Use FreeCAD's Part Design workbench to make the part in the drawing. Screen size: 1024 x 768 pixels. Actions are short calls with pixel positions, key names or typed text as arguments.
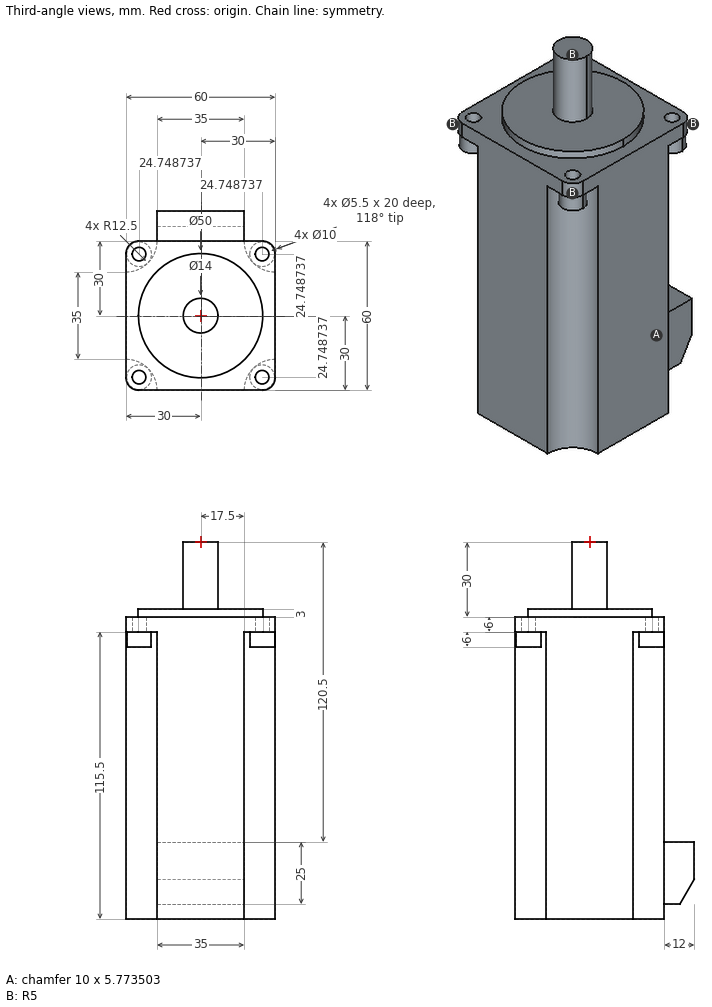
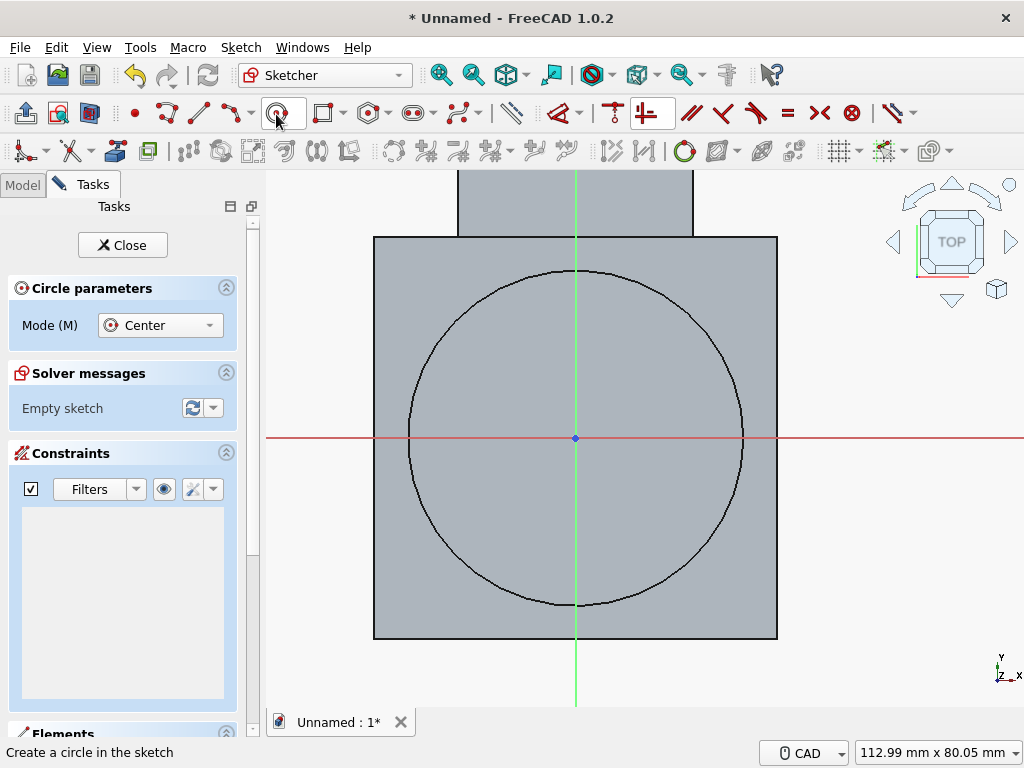
scroll(742, 272, up, 2)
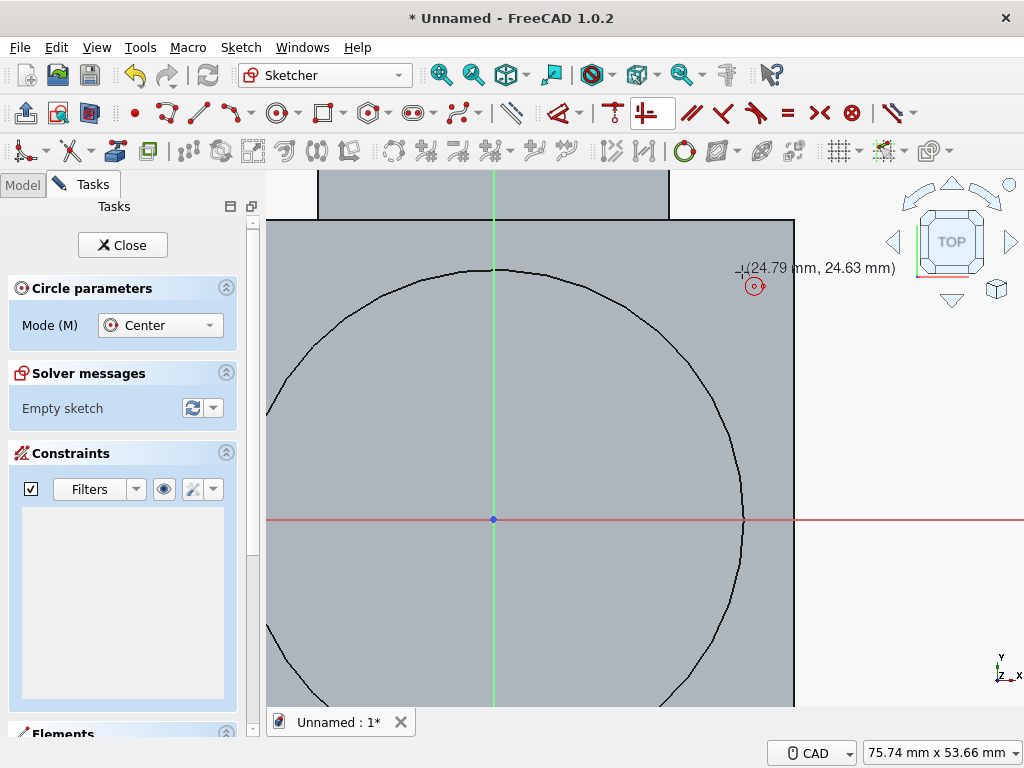
click(741, 272)
click(761, 253)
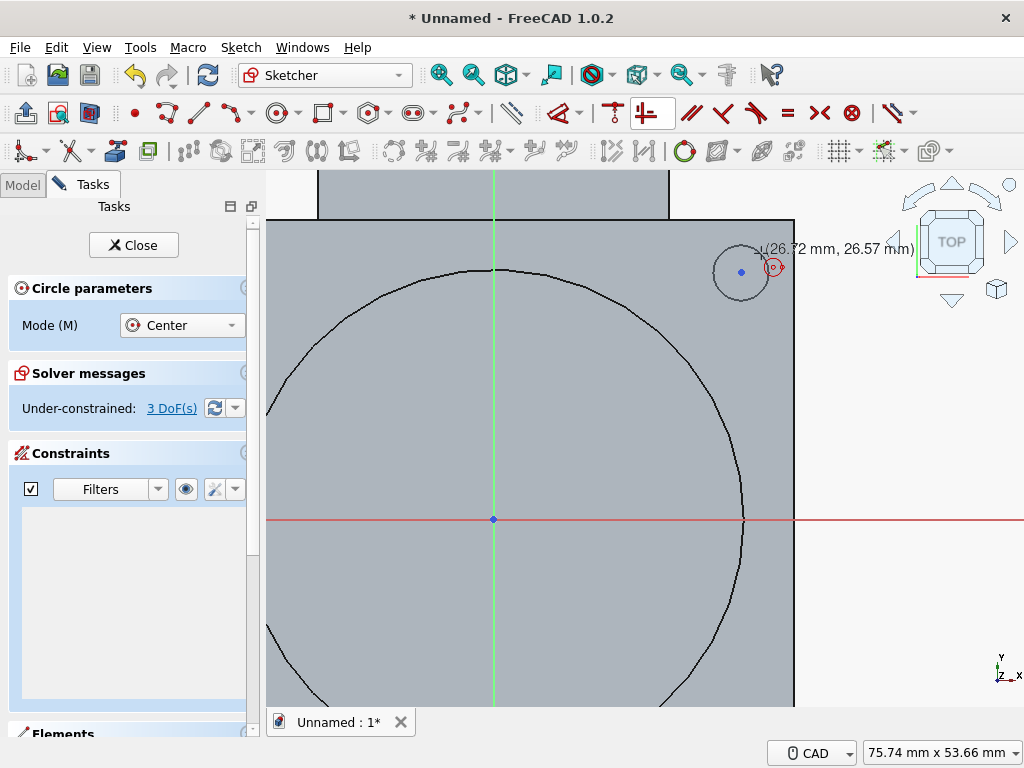
scroll(745, 273, down, 2)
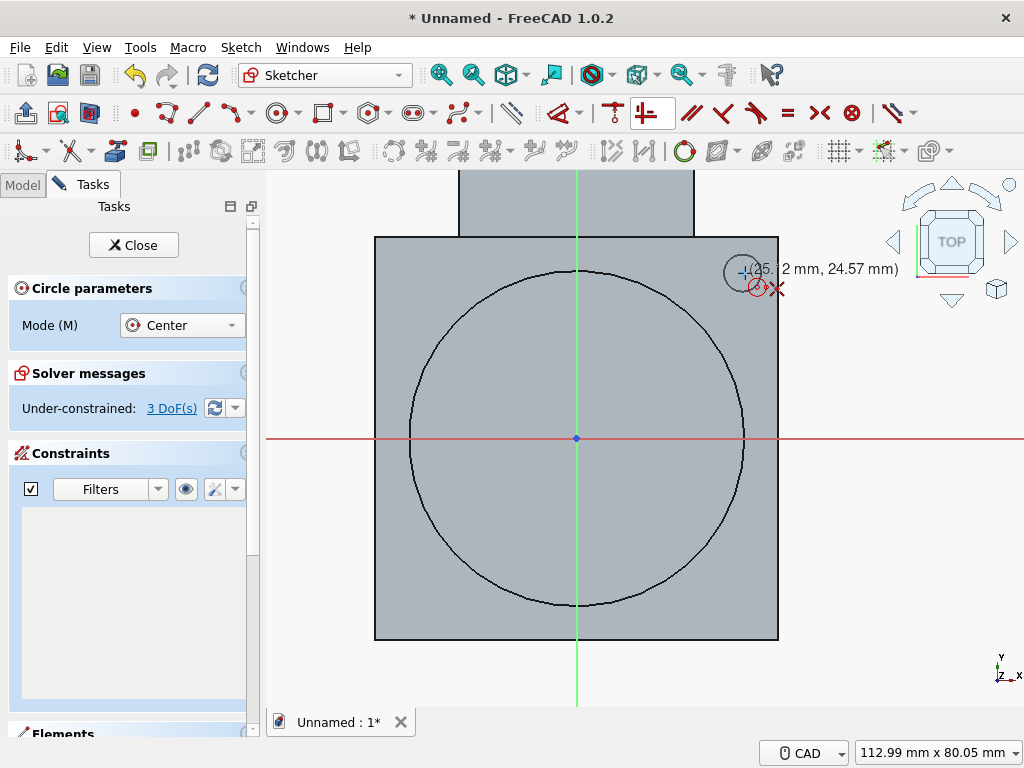
scroll(411, 273, up, 2)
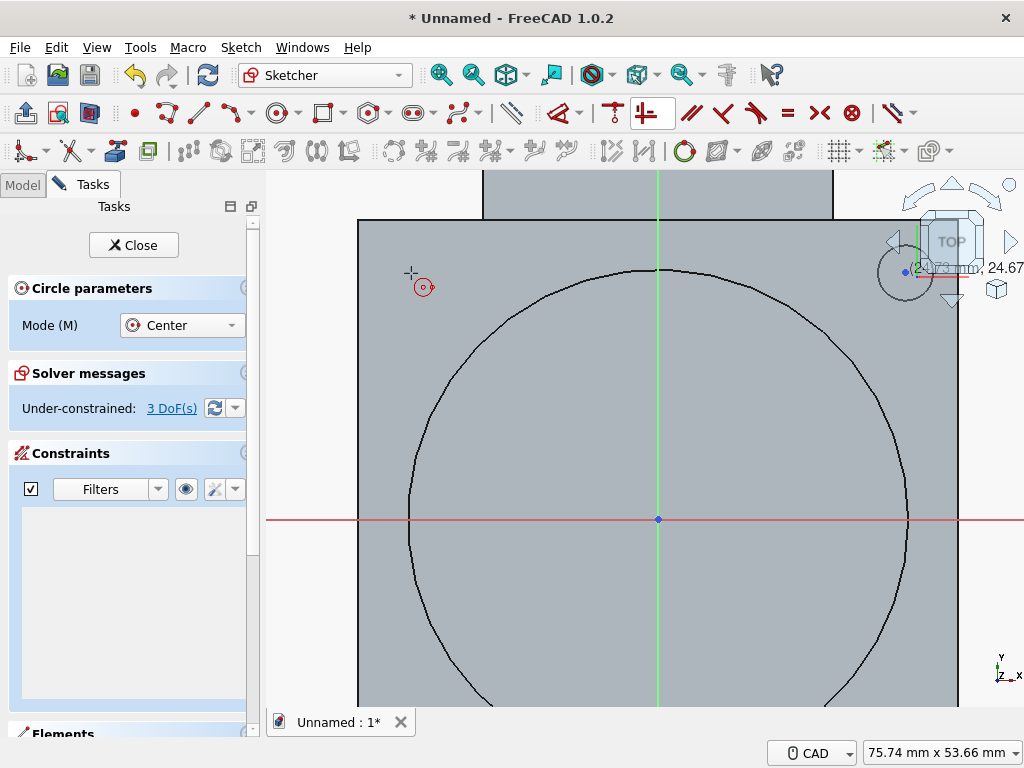
click(410, 272)
click(430, 253)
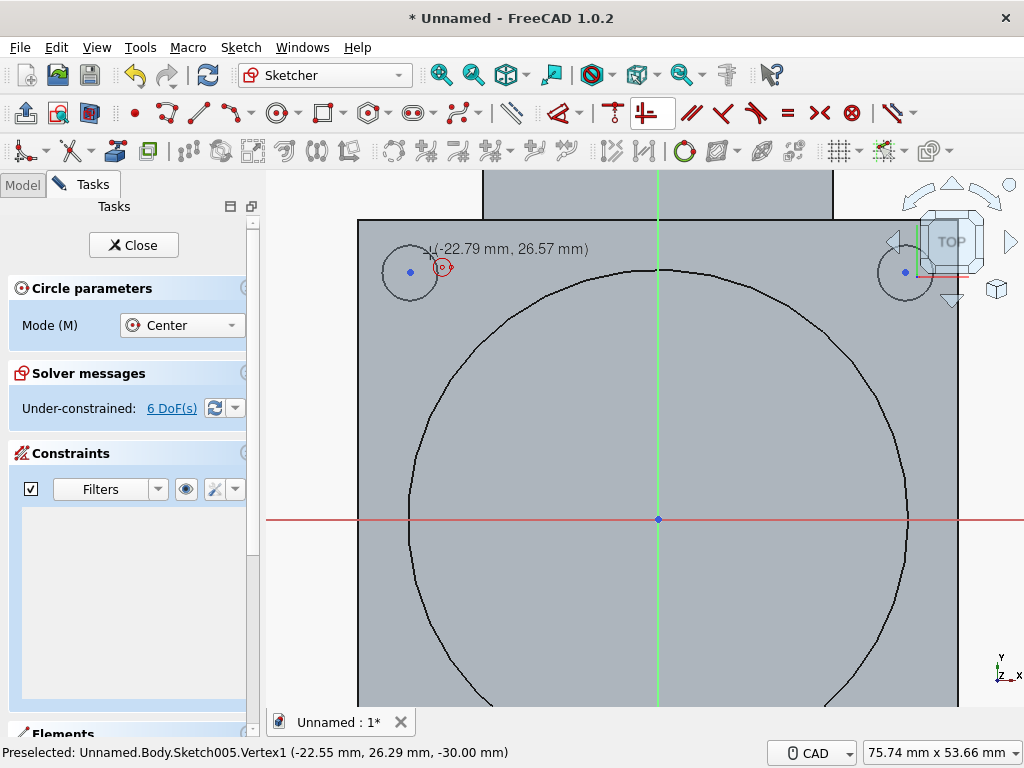
scroll(411, 273, down, 2)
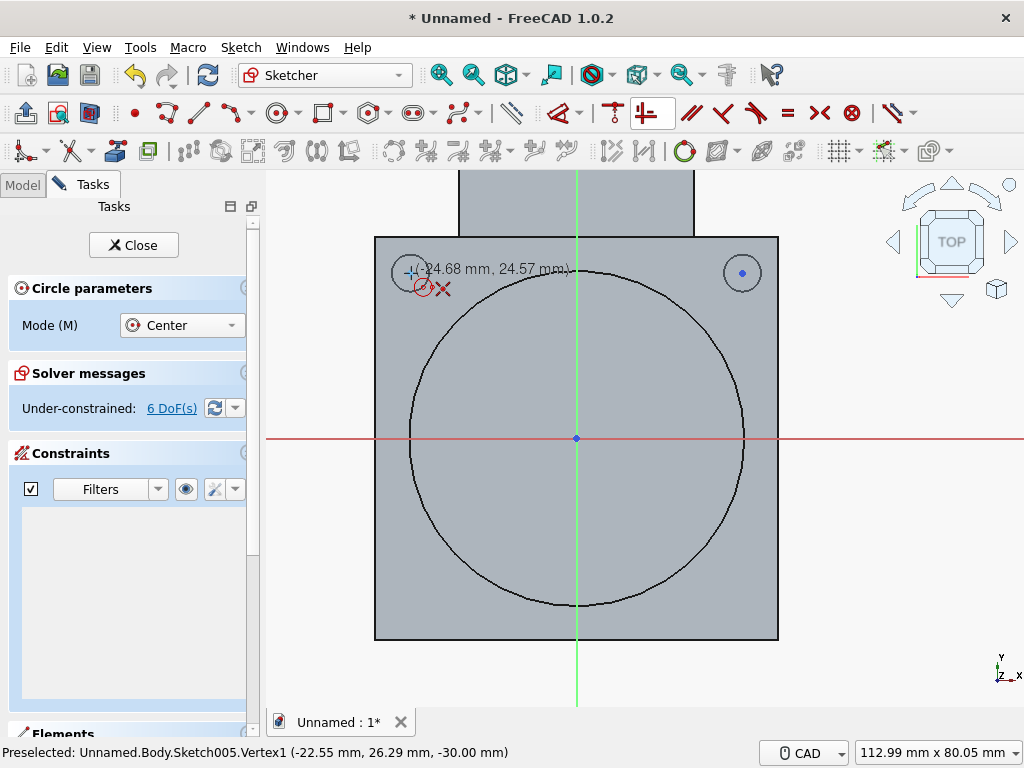
scroll(743, 605, up, 2)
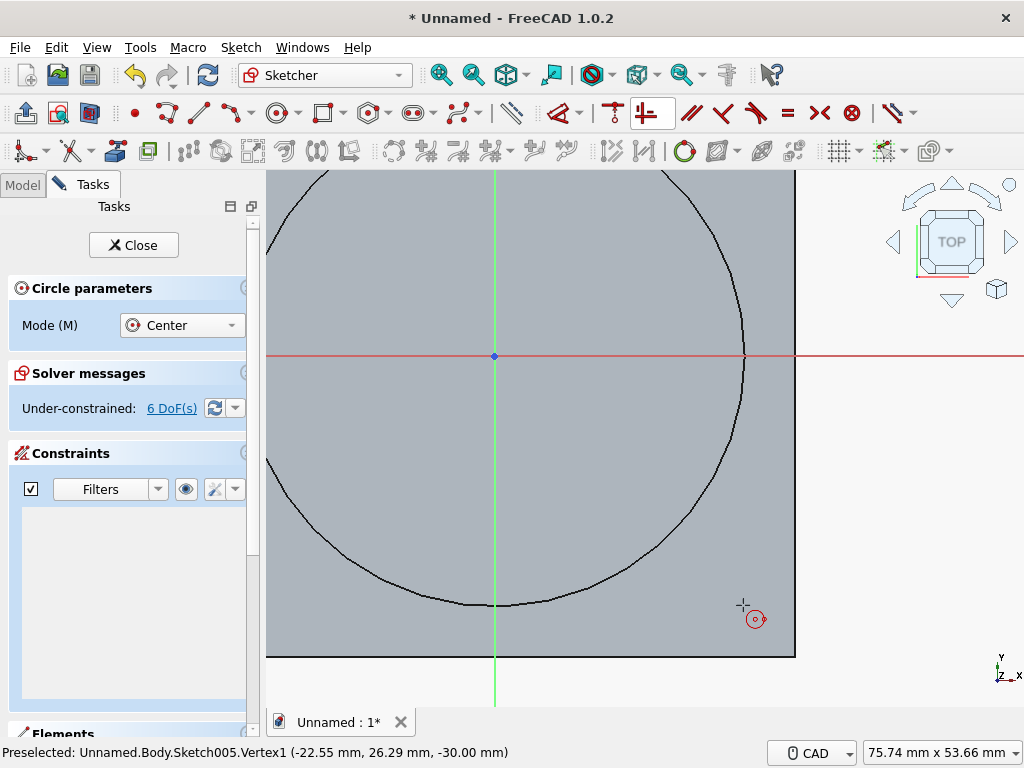
click(742, 604)
click(762, 585)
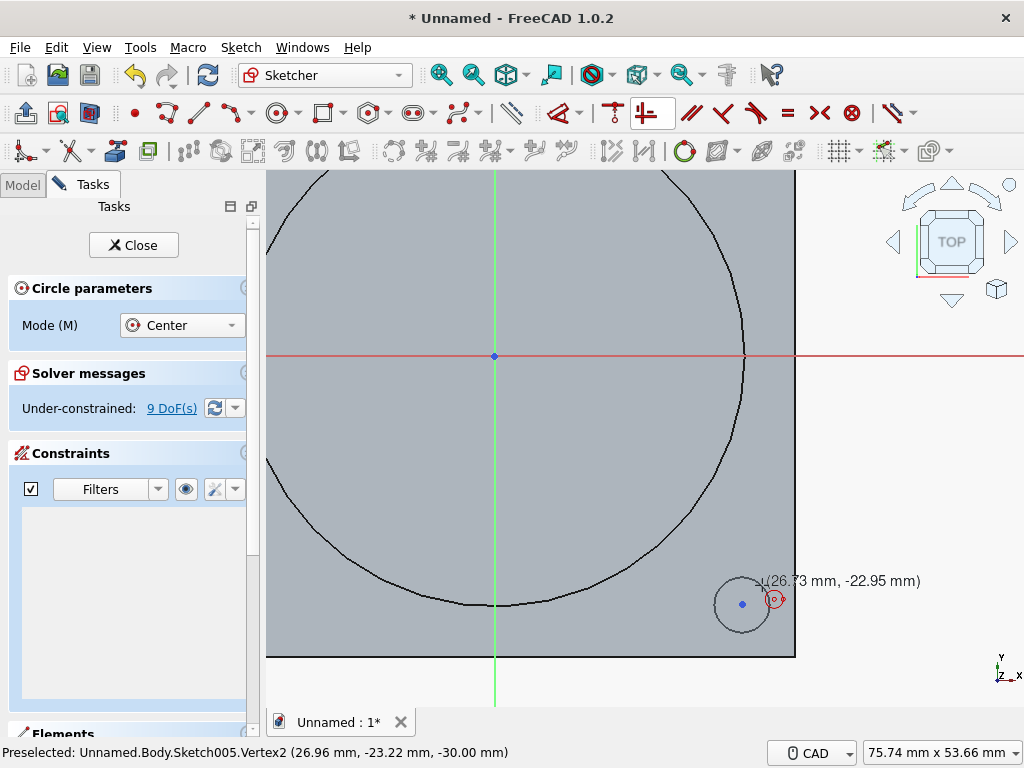
scroll(743, 606, down, 2)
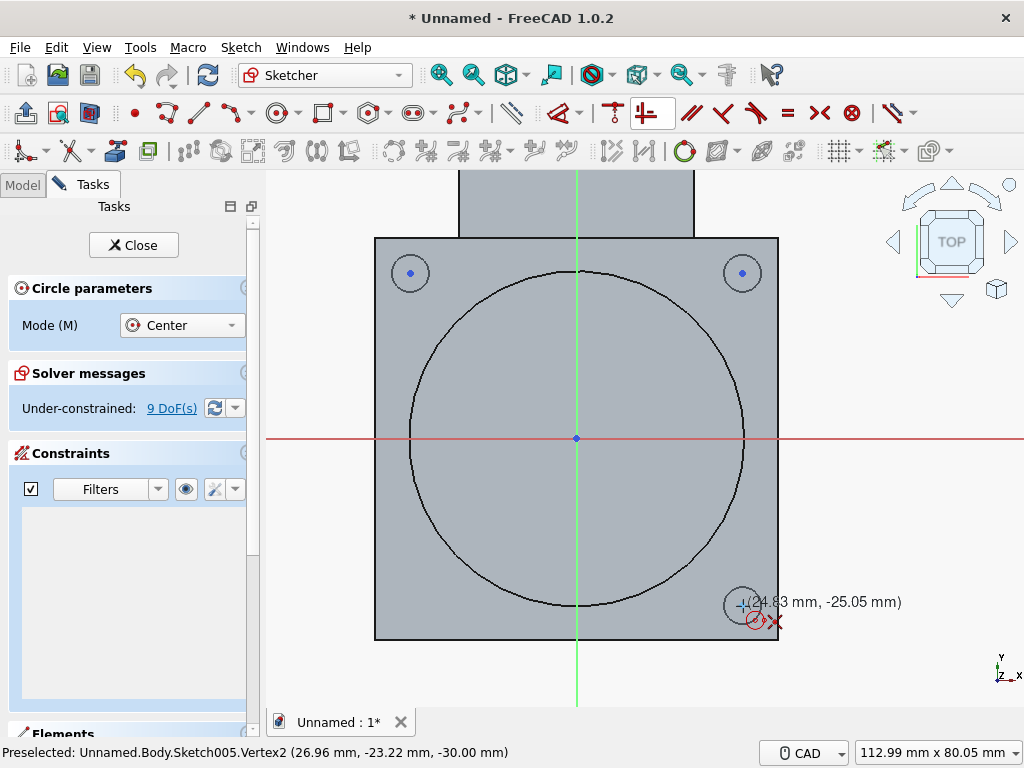
scroll(411, 605, up, 2)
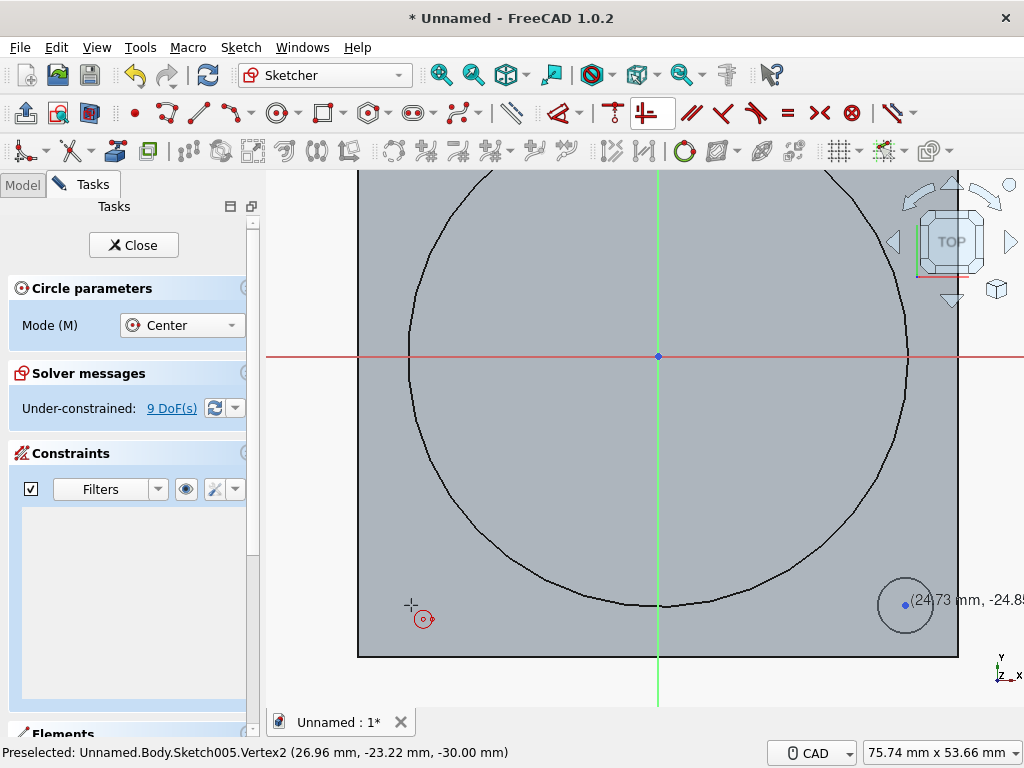
click(410, 604)
click(430, 585)
key(Escape)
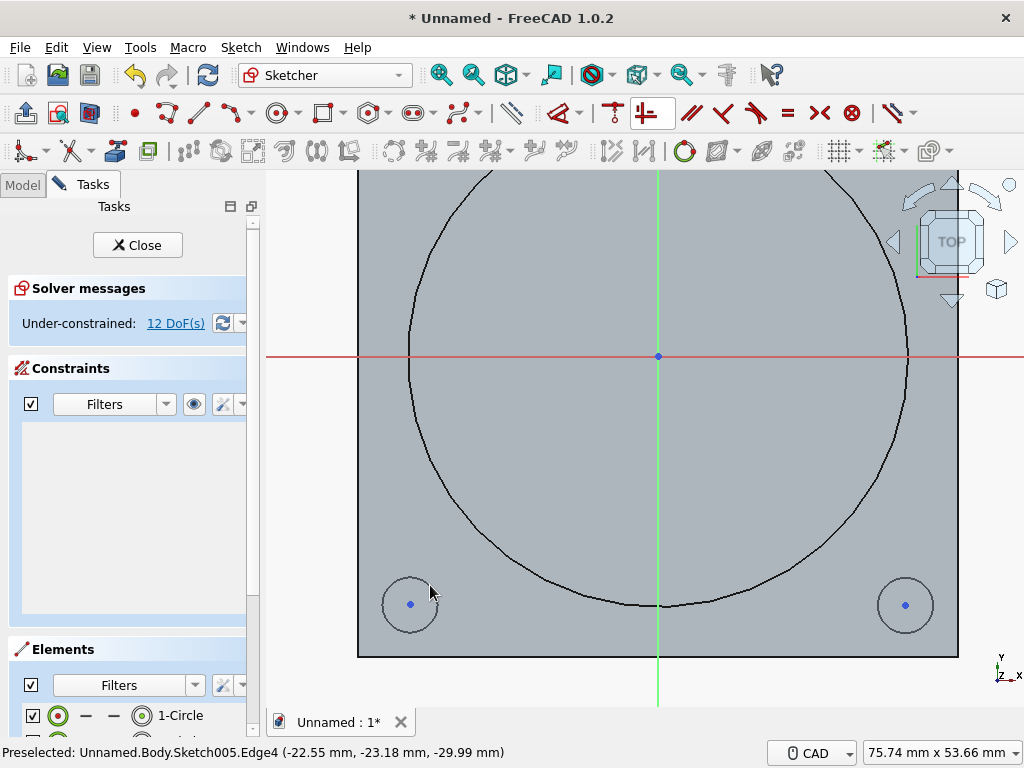
scroll(411, 605, down, 2)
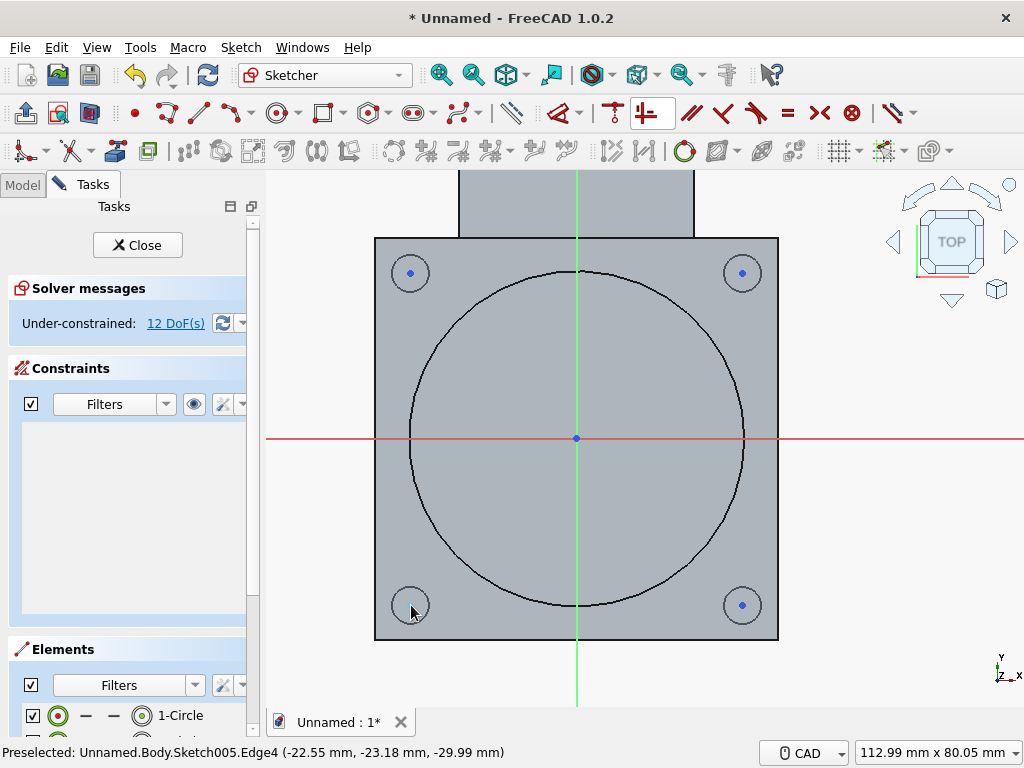
click(756, 260)